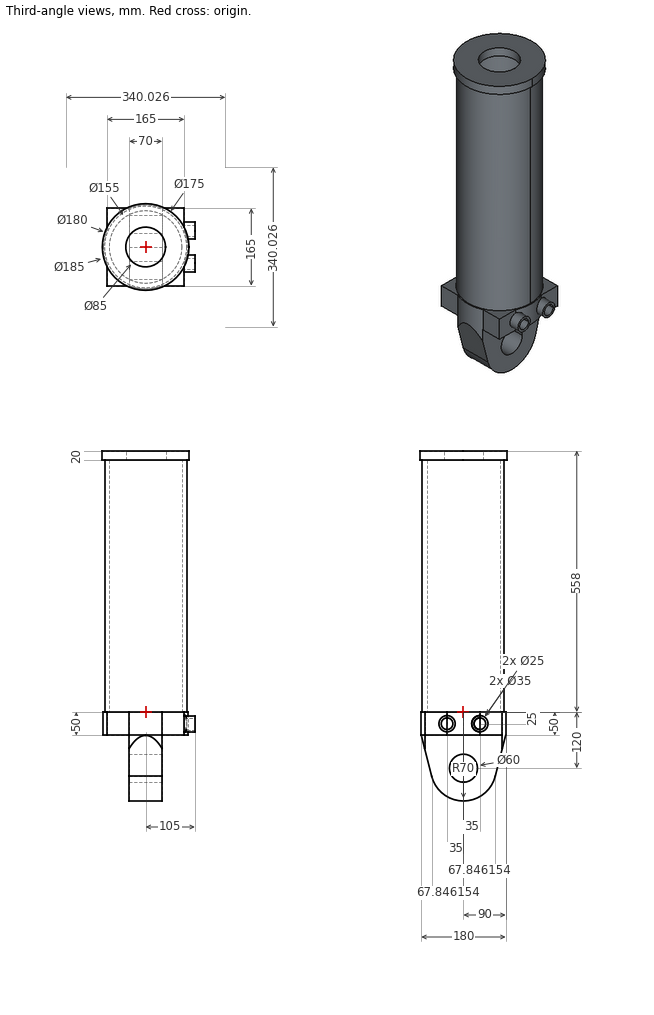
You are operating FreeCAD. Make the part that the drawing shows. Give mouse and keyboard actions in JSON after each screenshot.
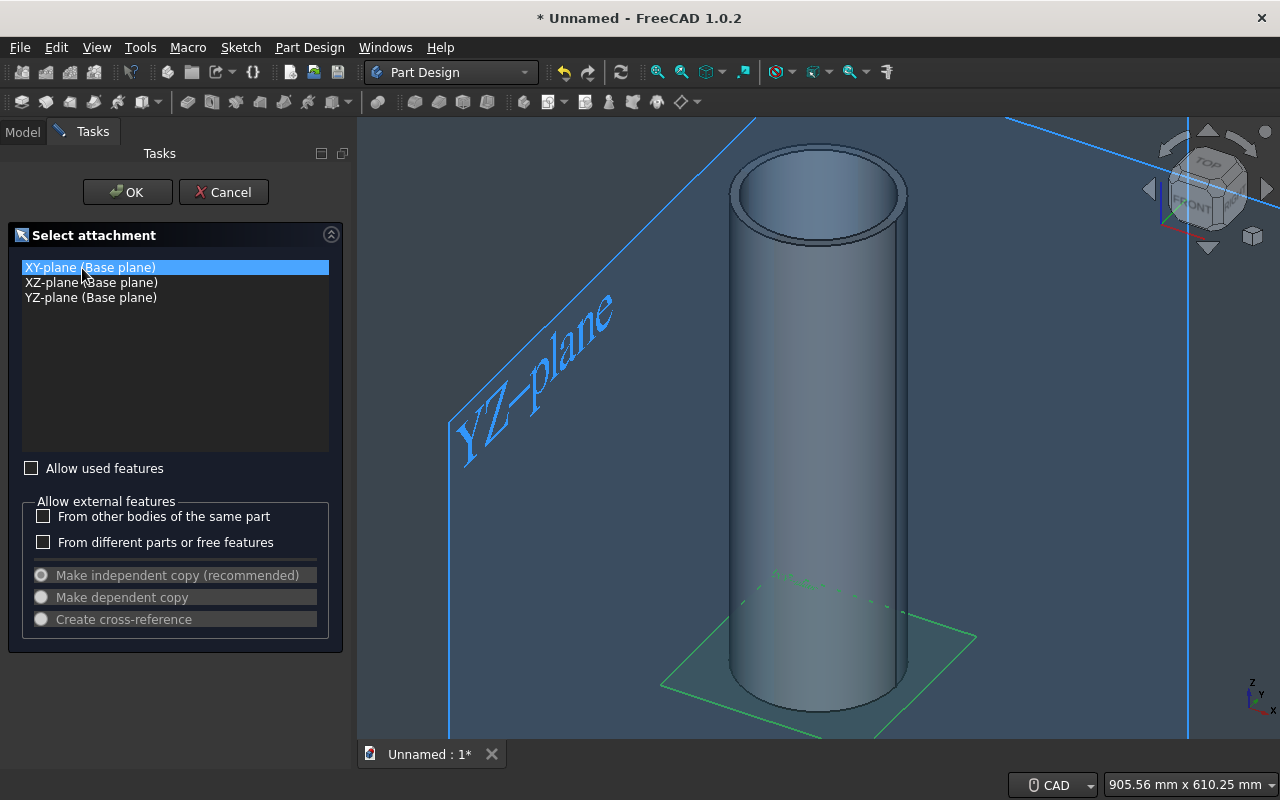
{"action": "left_click", "coordinate": [128, 192]}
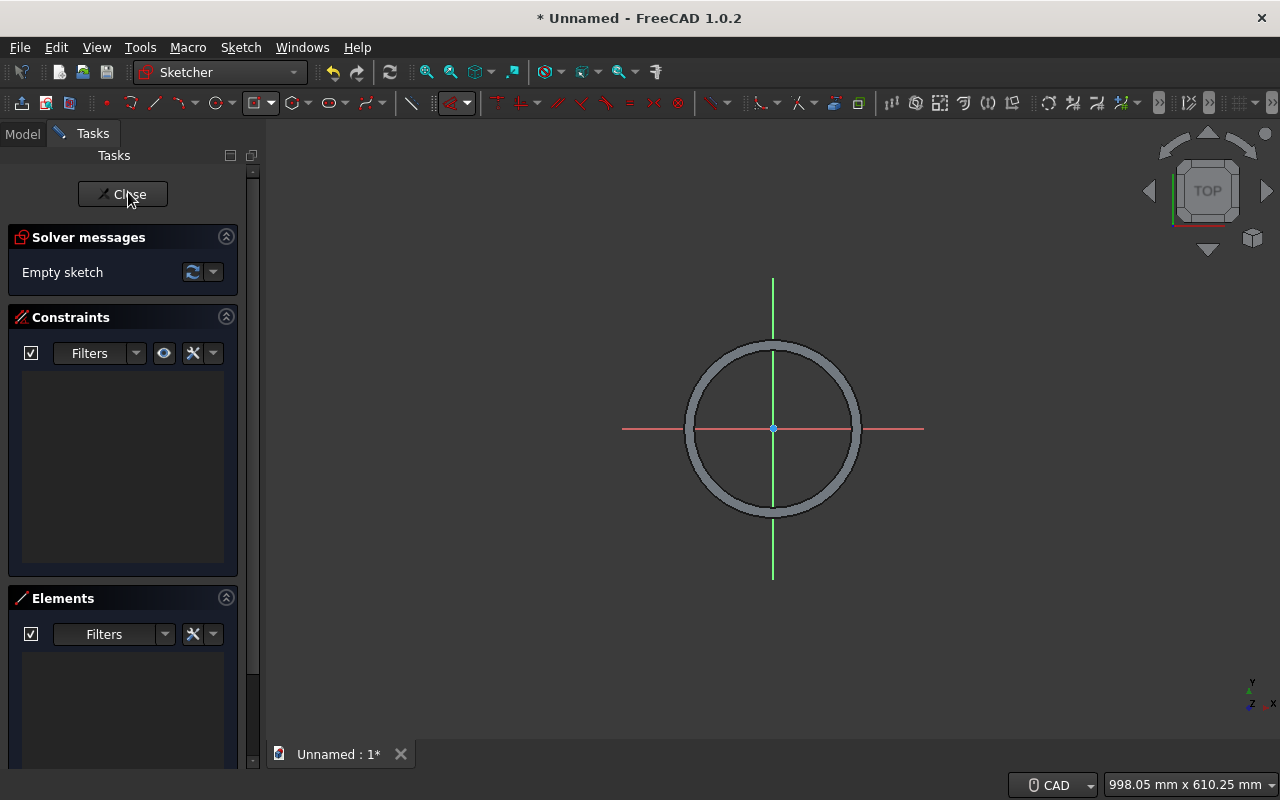
{"action": "left_click", "coordinate": [70, 104]}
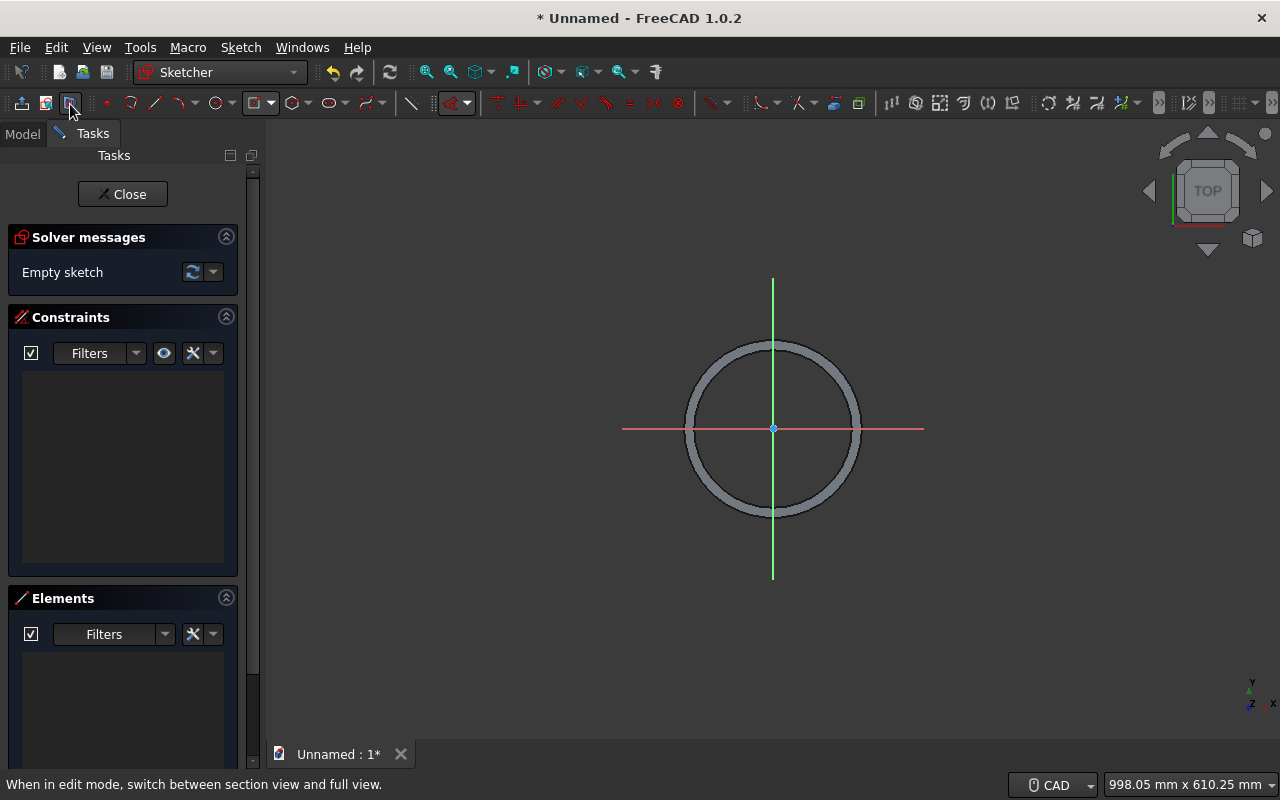
{"action": "scroll", "coordinate": [829, 429], "scroll_direction": "up", "scroll_amount": 4}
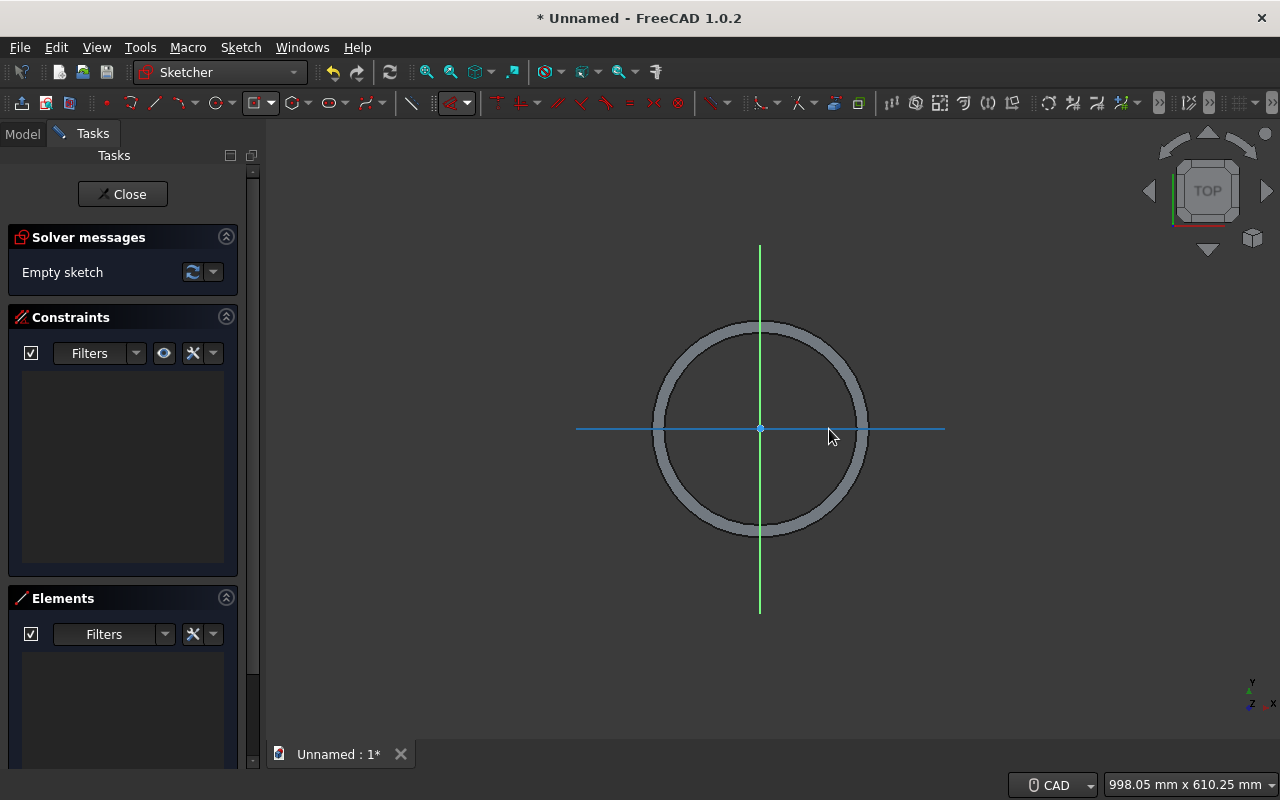
{"action": "left_click", "coordinate": [216, 104]}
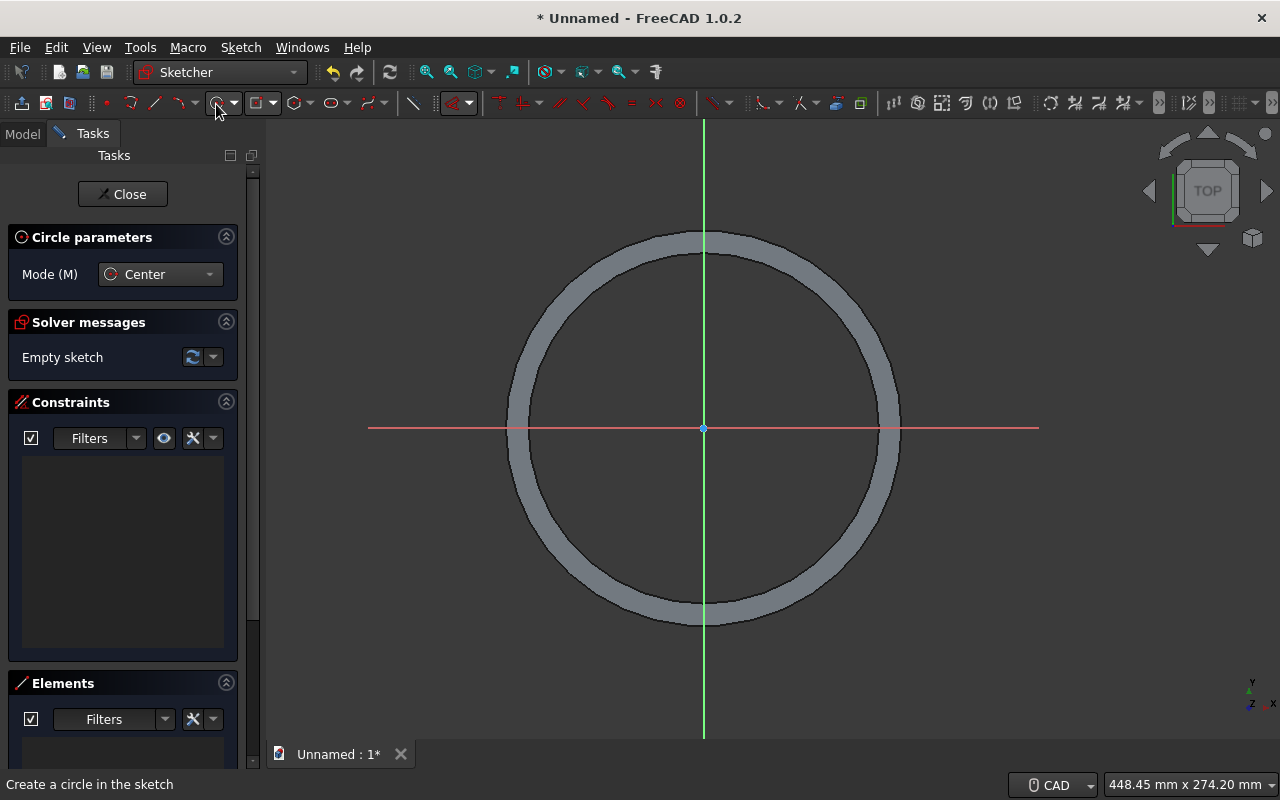
{"action": "left_click", "coordinate": [704, 428]}
{"action": "left_click", "coordinate": [848, 284]}
{"action": "key", "text": "Escape"}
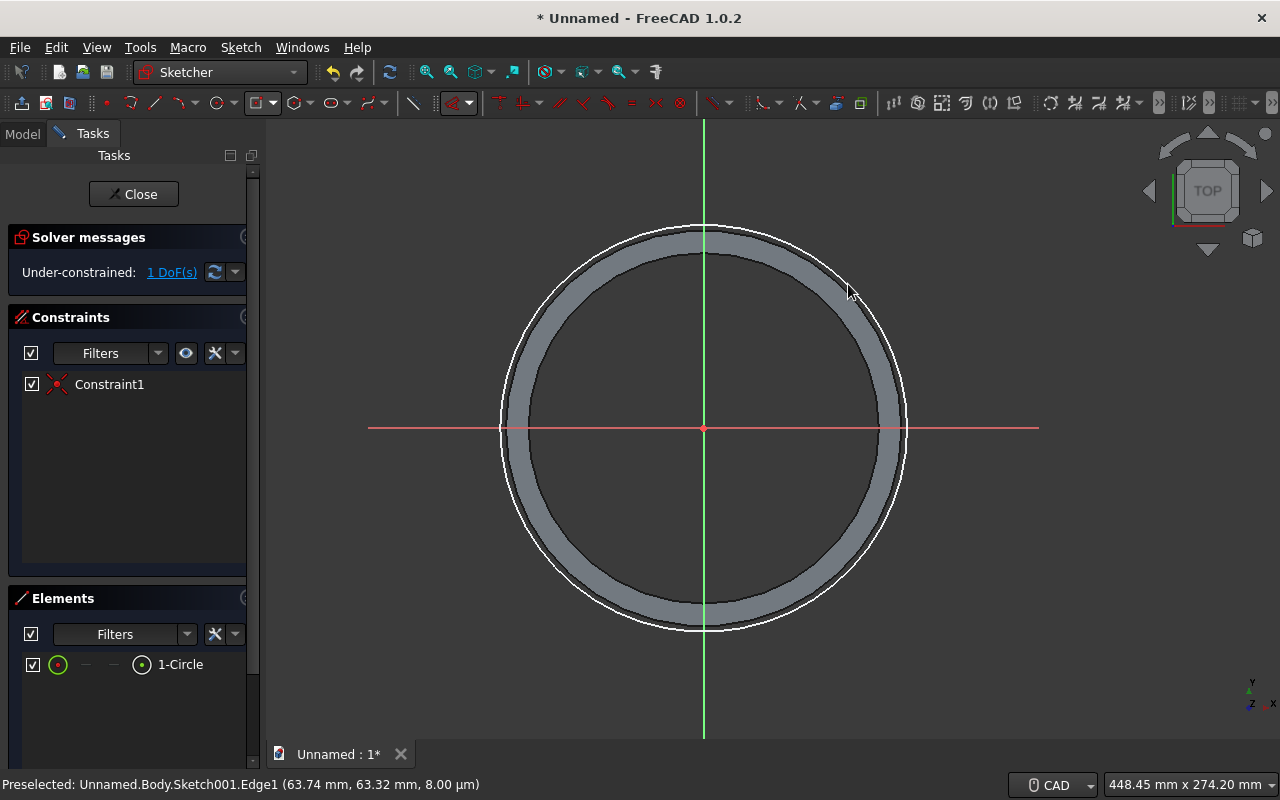
{"action": "left_click", "coordinate": [452, 104]}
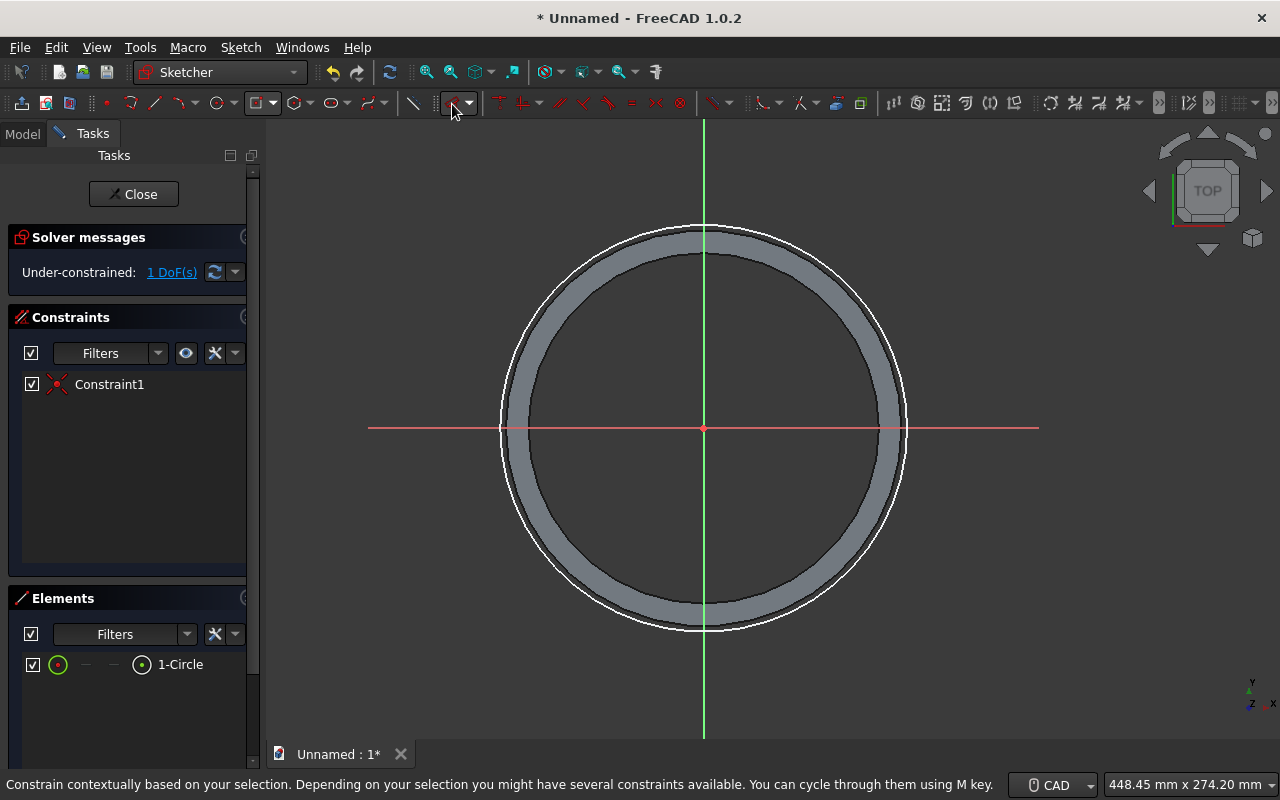
{"action": "left_click", "coordinate": [847, 284]}
{"action": "left_click", "coordinate": [870, 261]}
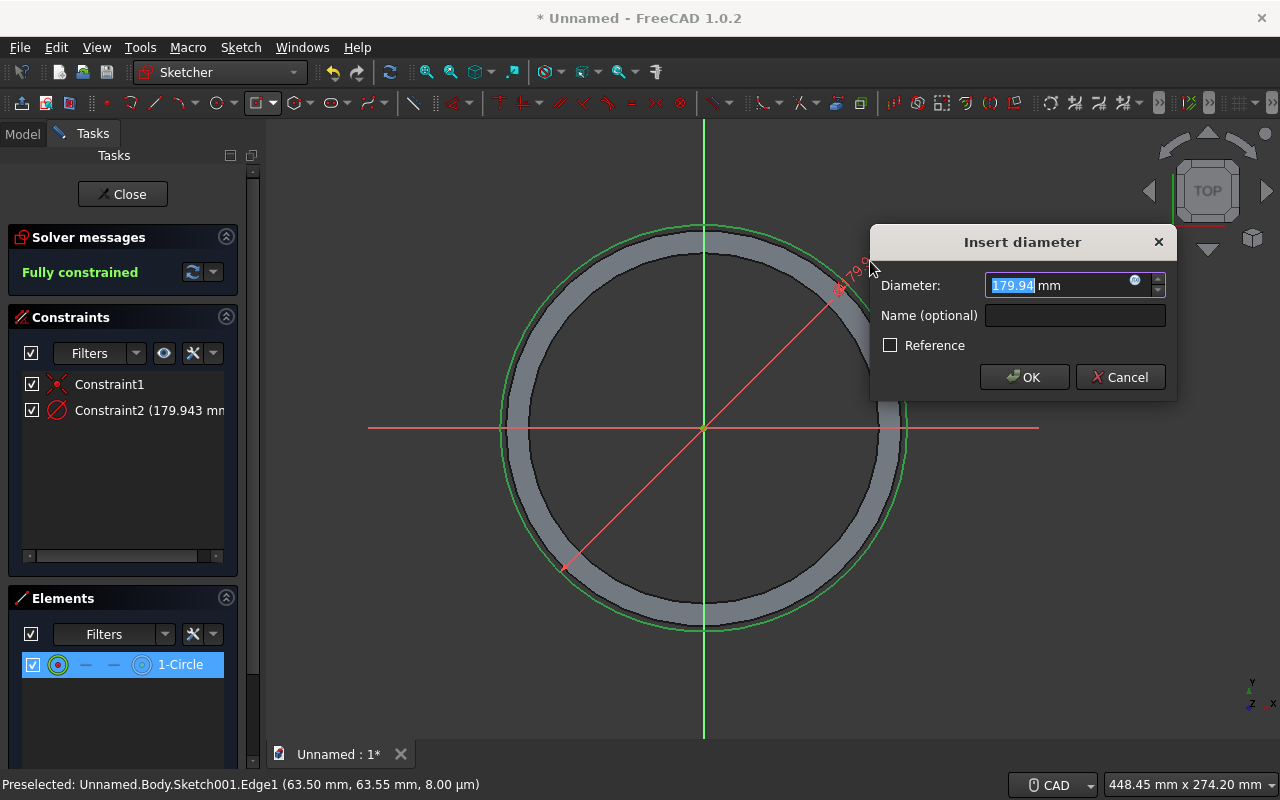
{"action": "type", "text": "180"}
{"action": "key", "text": "Return"}
{"action": "key", "text": "Escape"}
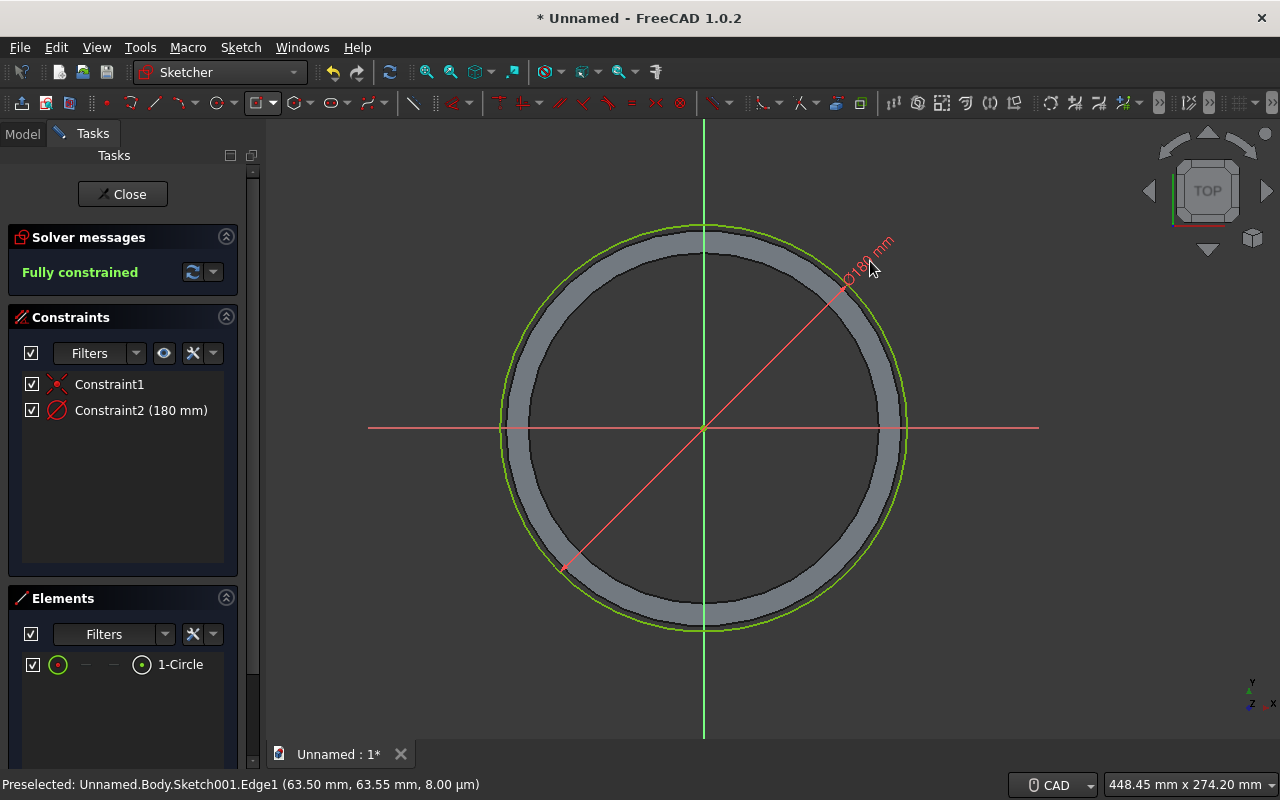
{"action": "left_click", "coordinate": [123, 194]}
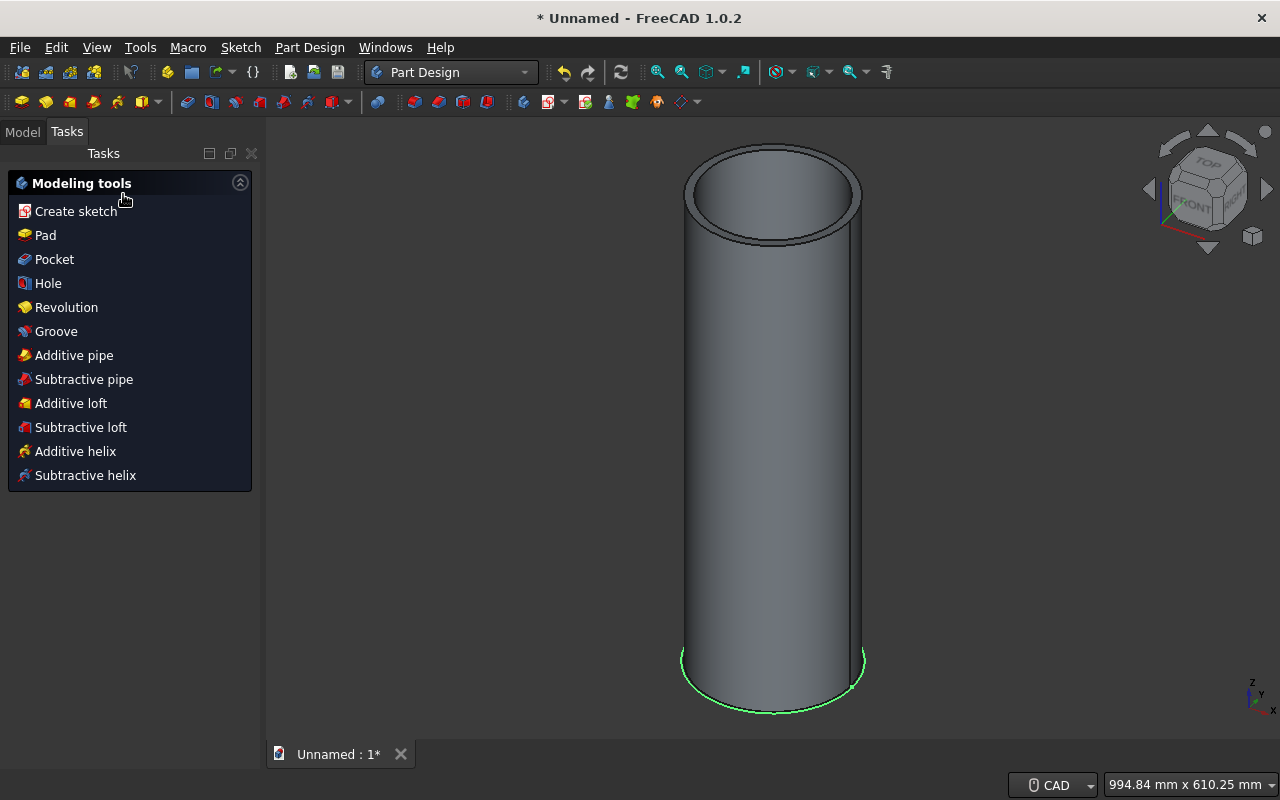
{"action": "left_click", "coordinate": [22, 102]}